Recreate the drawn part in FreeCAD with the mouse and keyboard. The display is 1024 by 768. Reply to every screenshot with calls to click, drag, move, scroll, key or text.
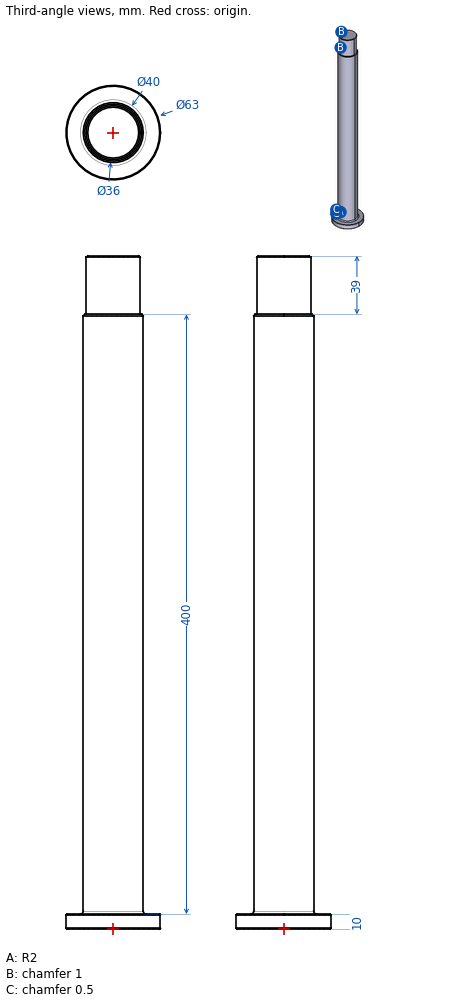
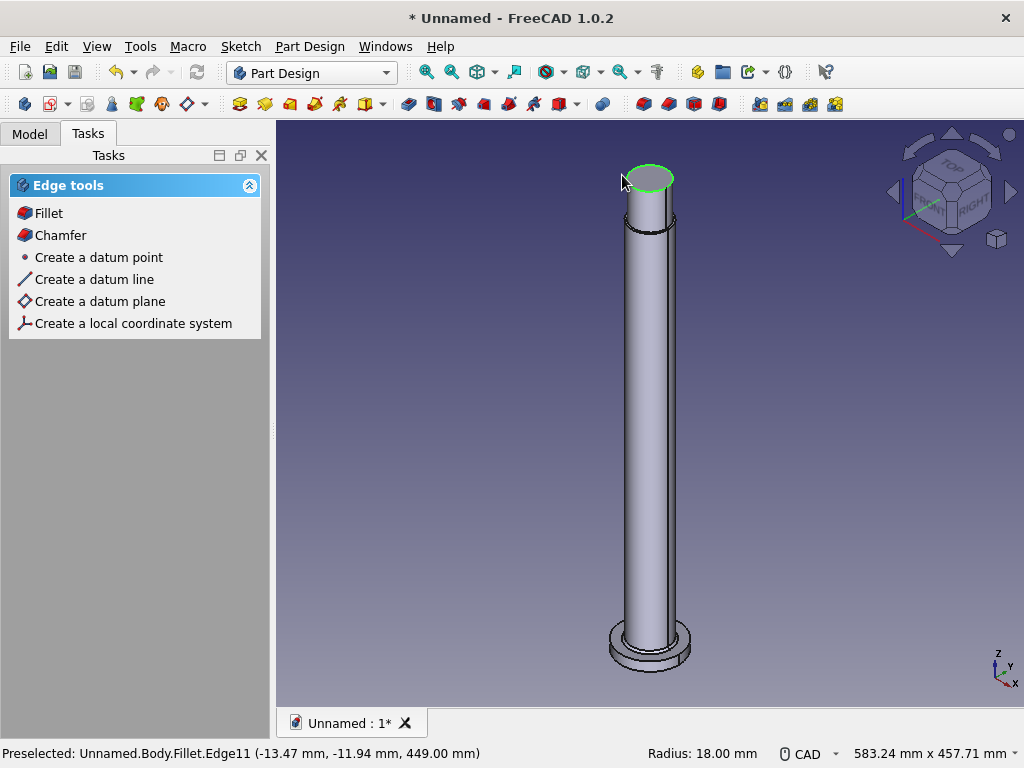
click(627, 225, ctrl)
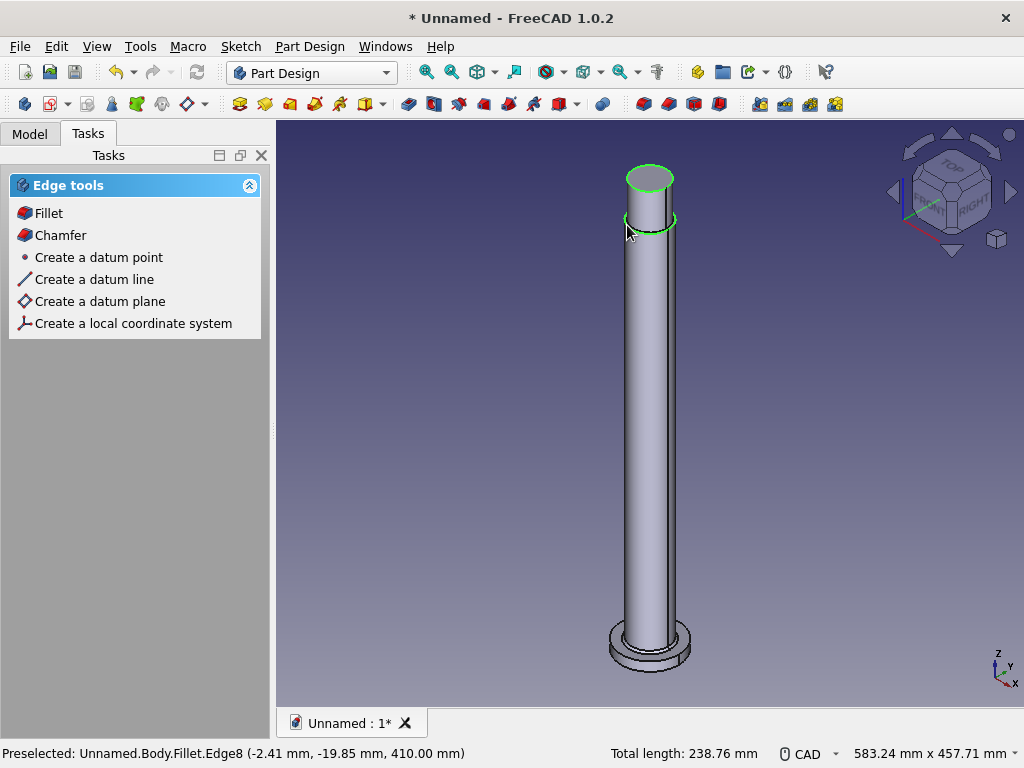
click(669, 104)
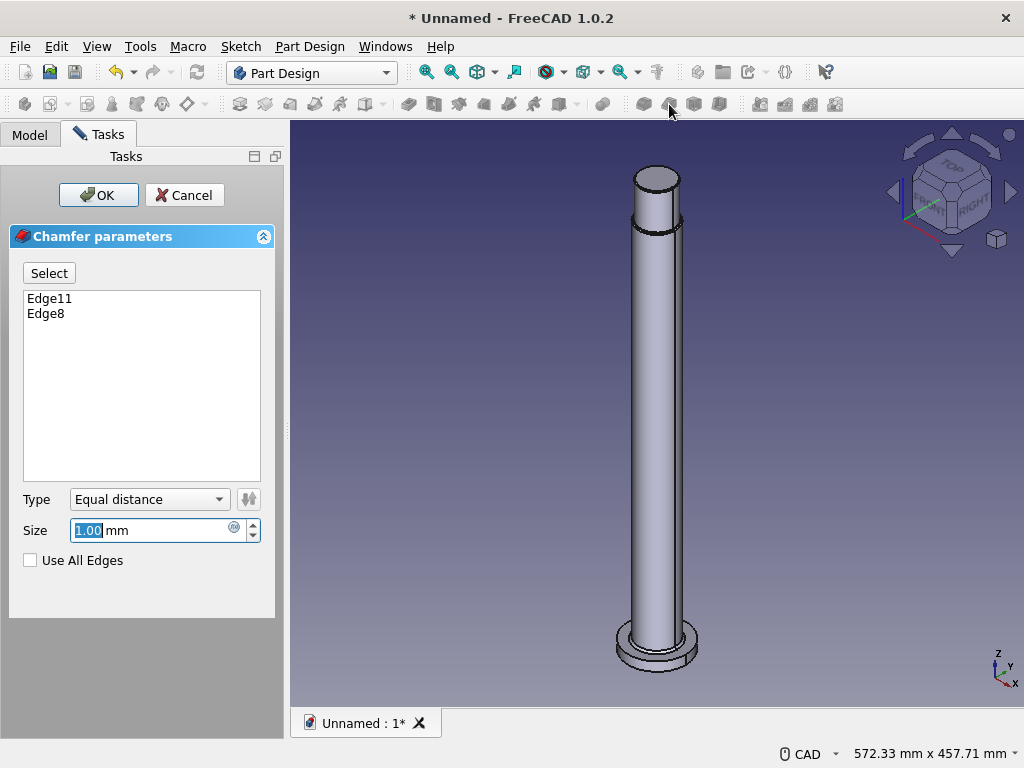
text(1)
key(Tab)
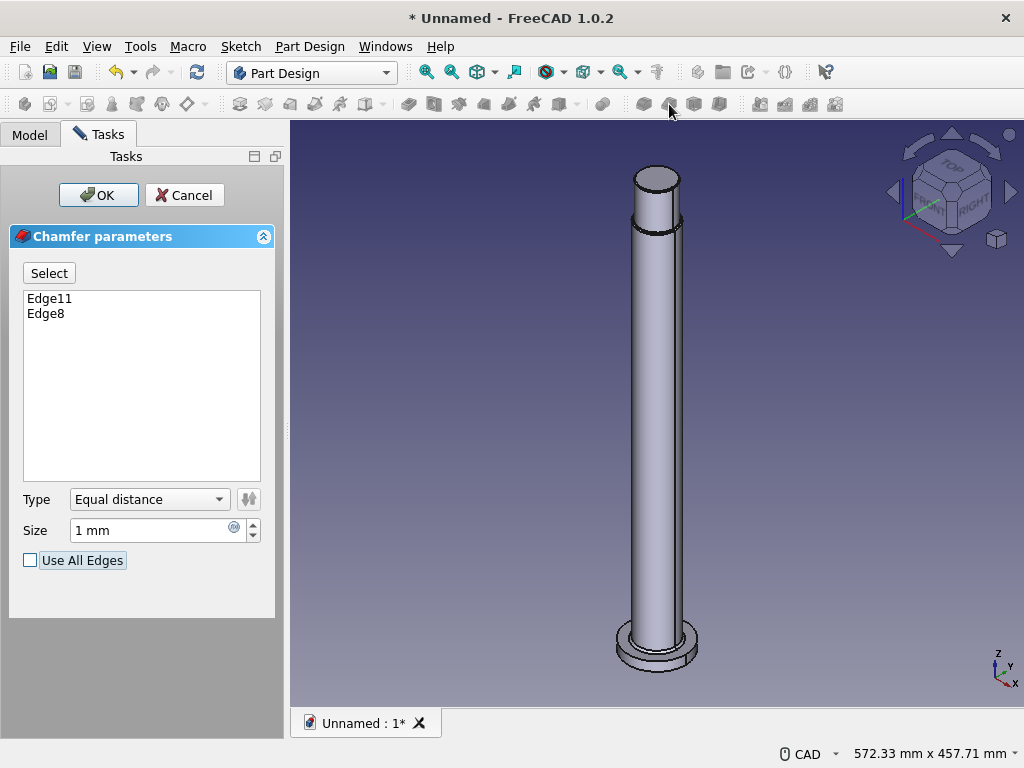
click(99, 195)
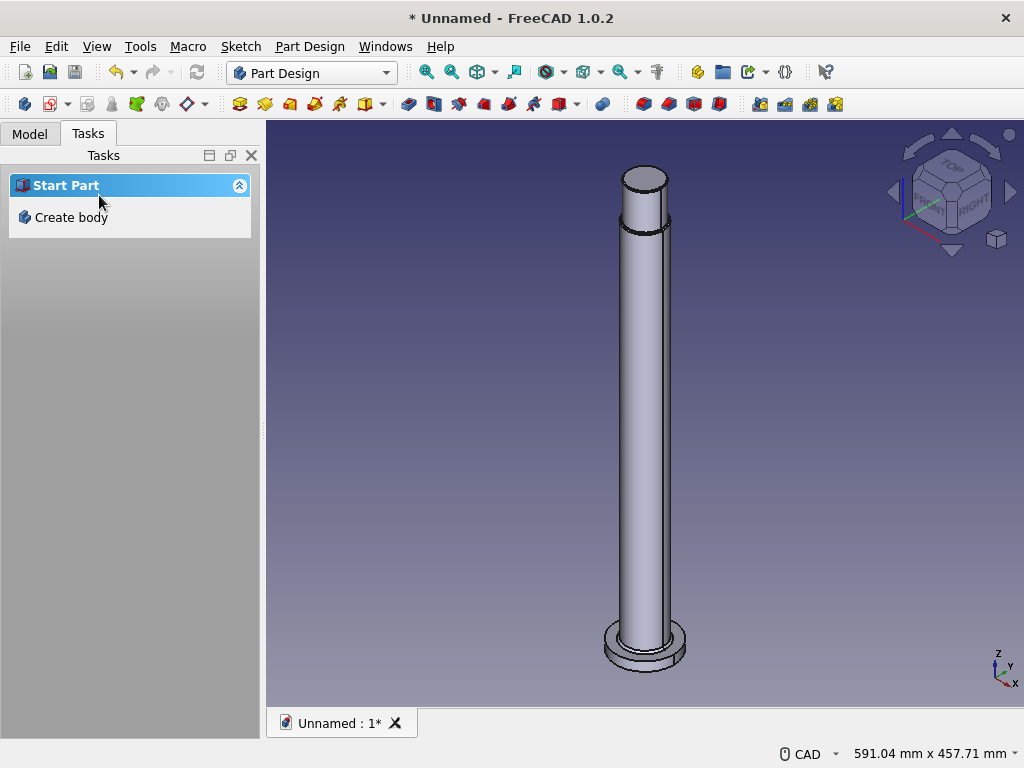
click(609, 648)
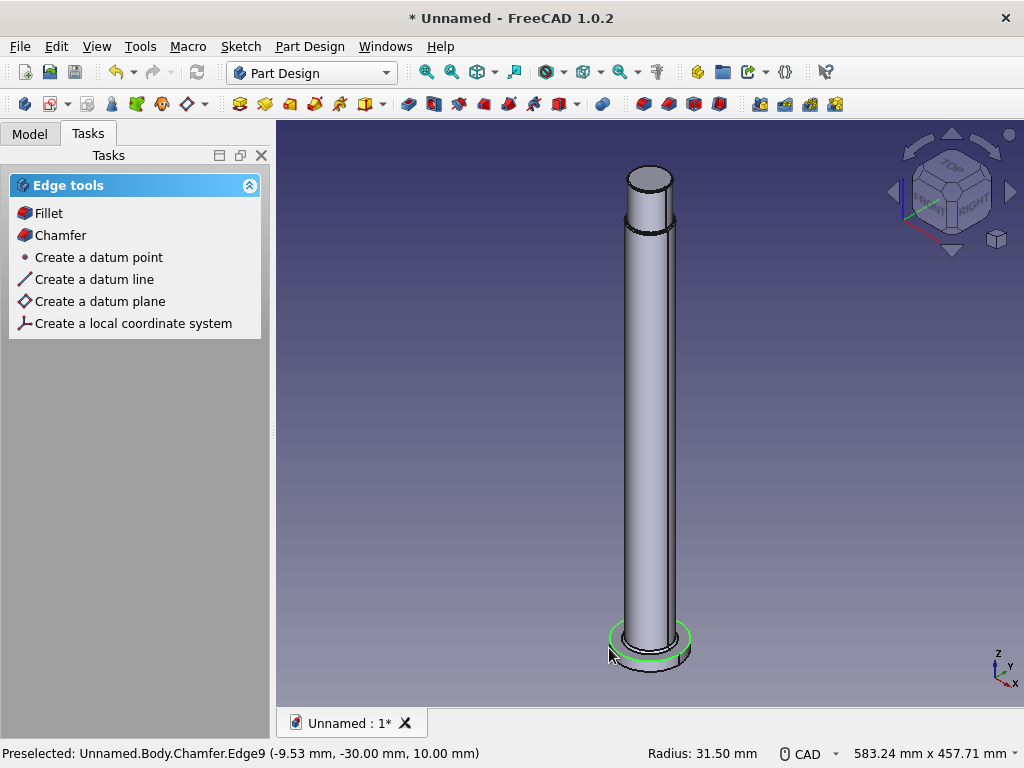
key(2)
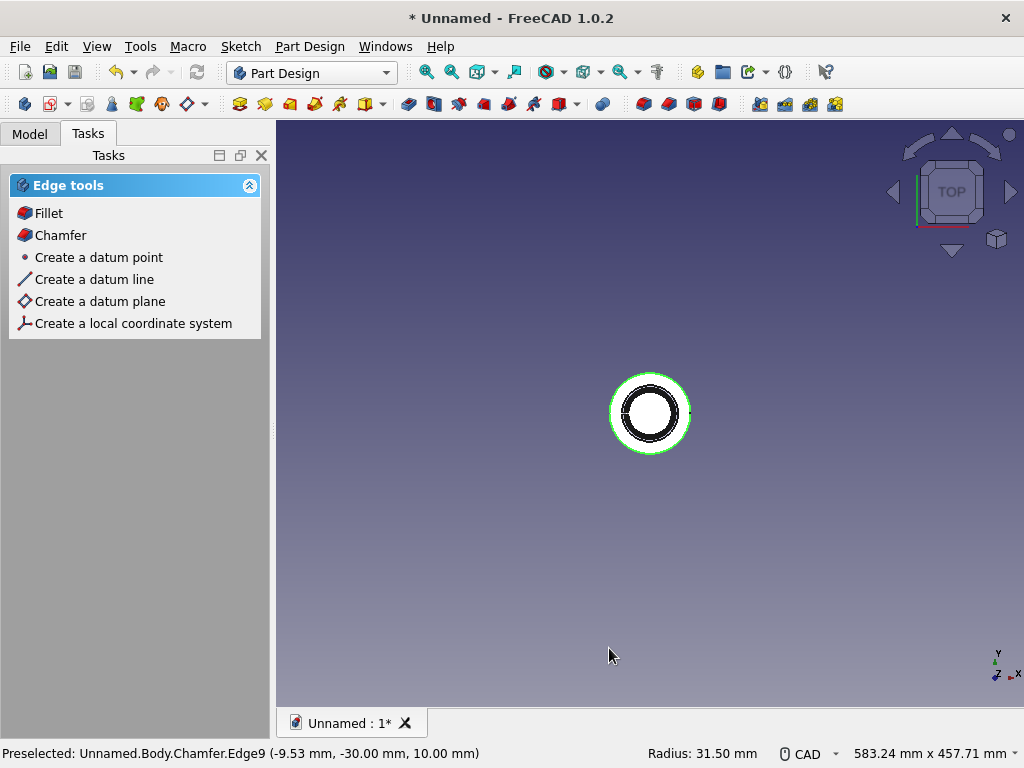
click(427, 72)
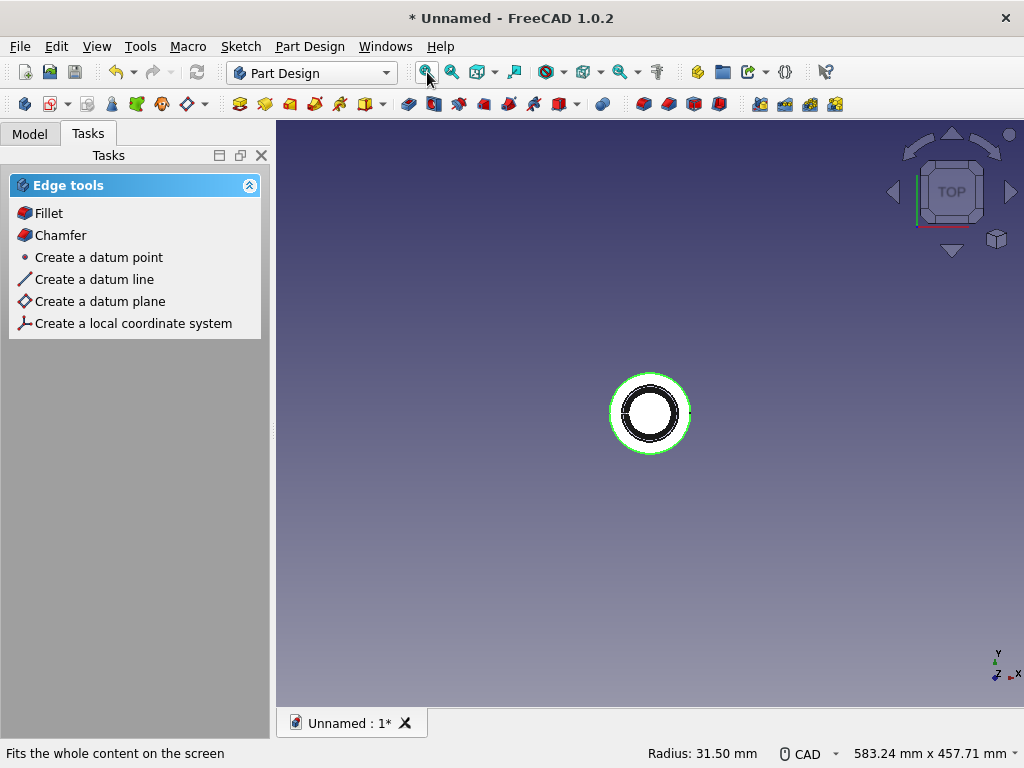
key(0)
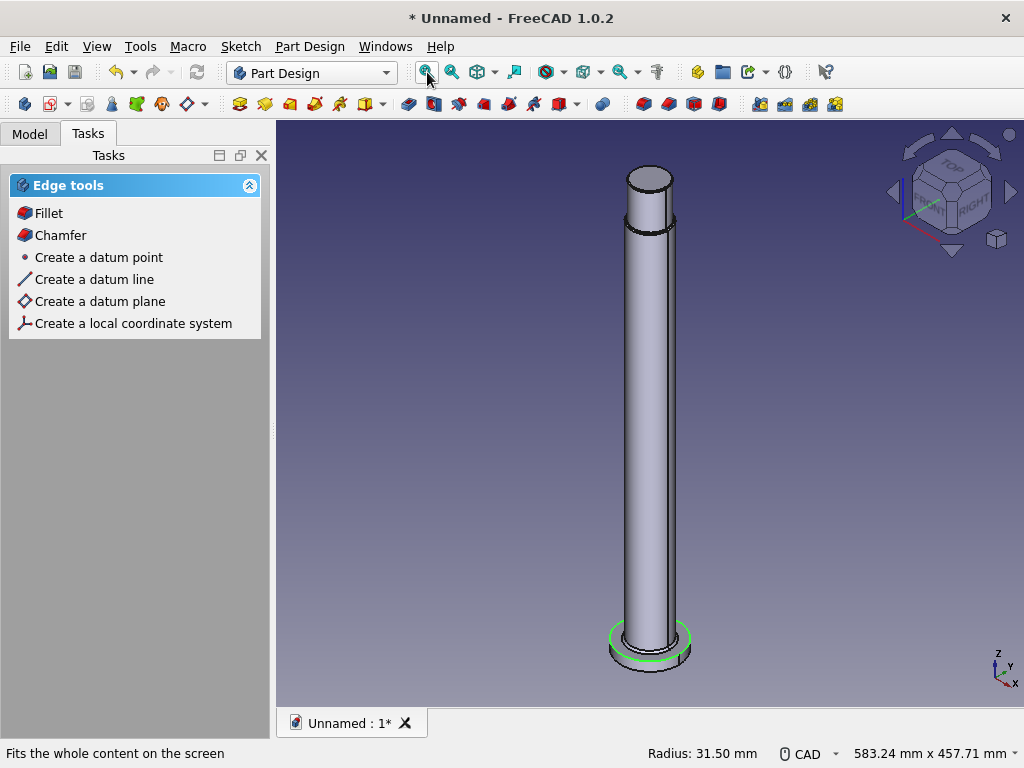
key(1)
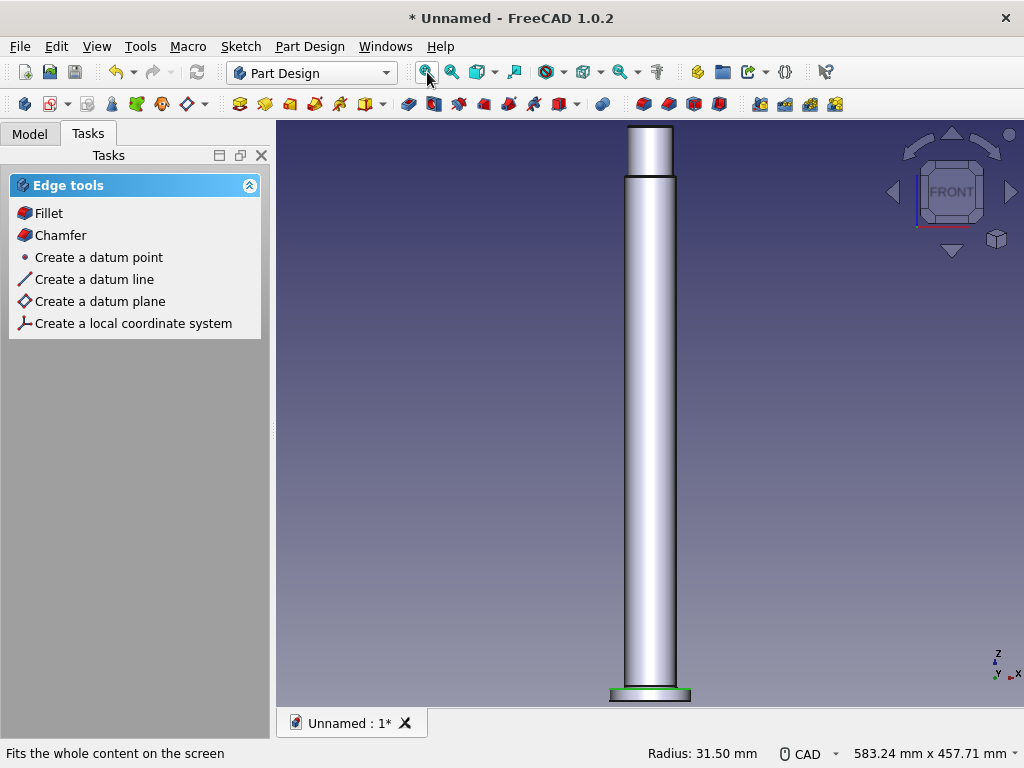
key(3)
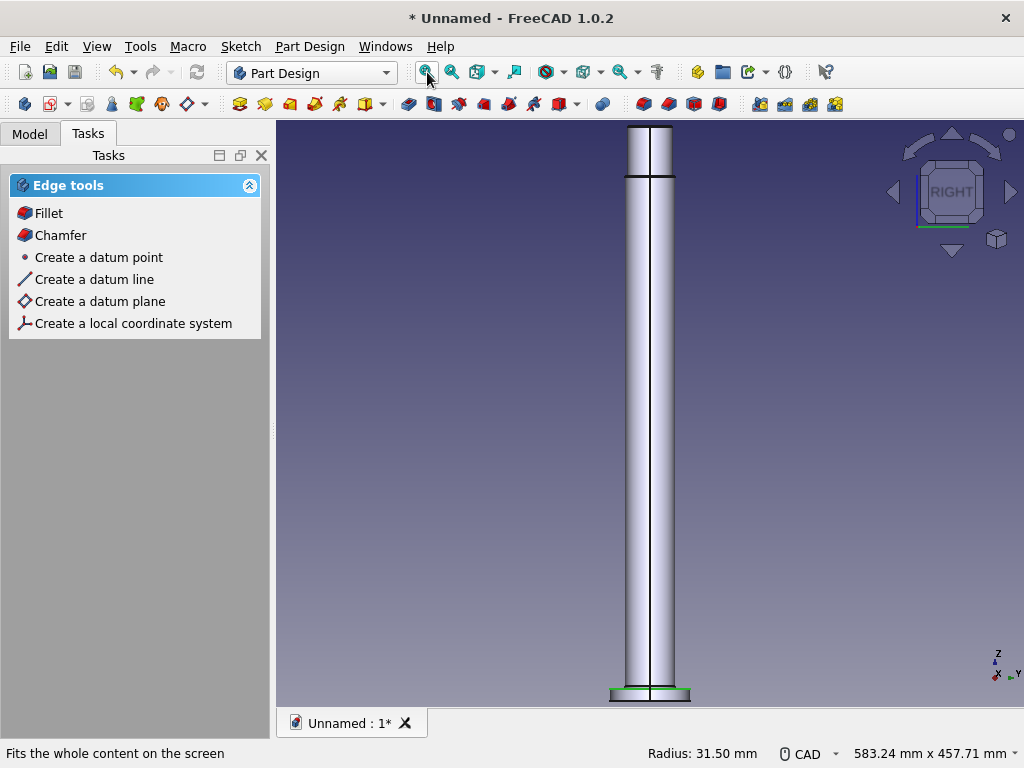
key(5)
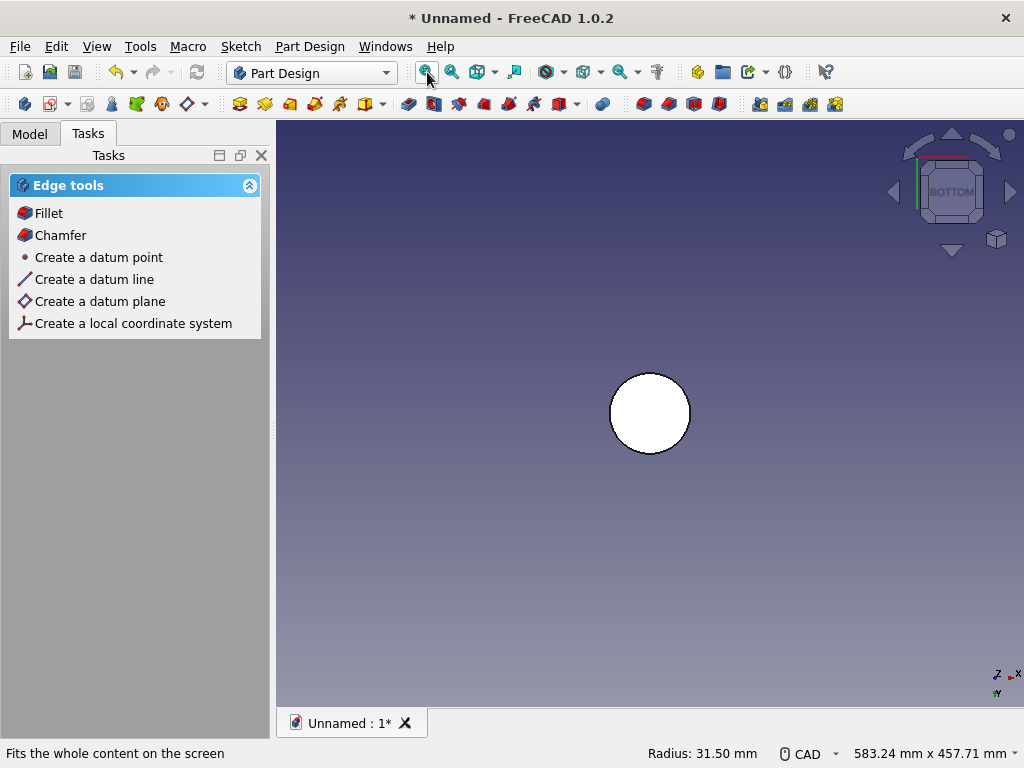
click(427, 72)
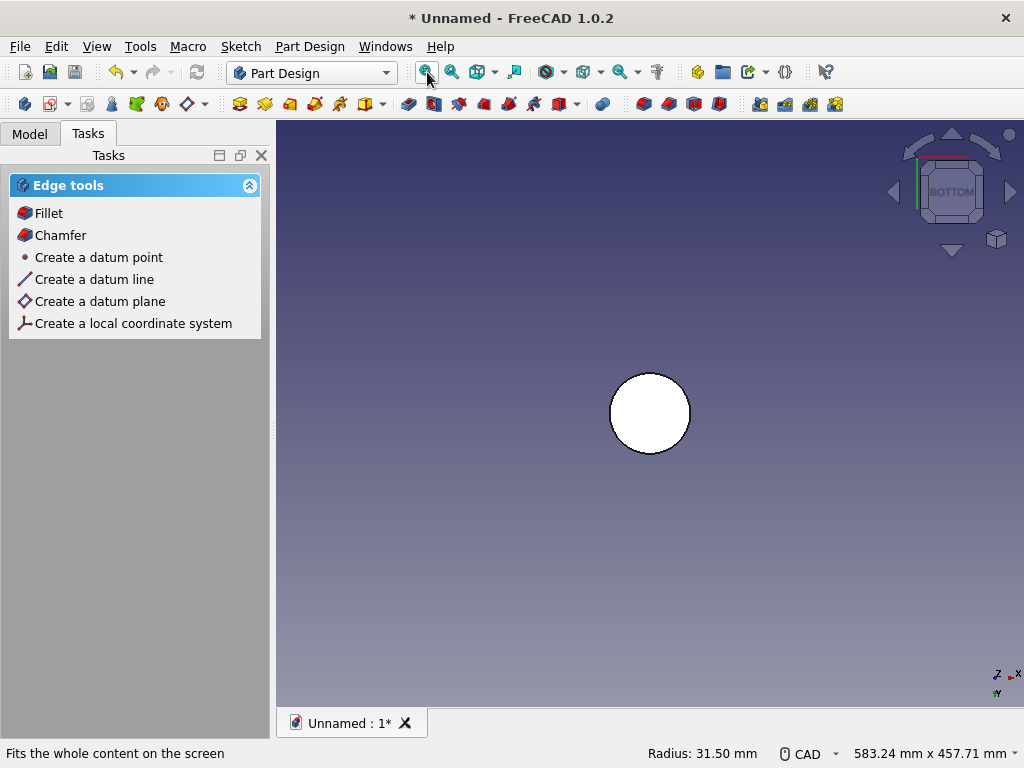
click(617, 436, ctrl)